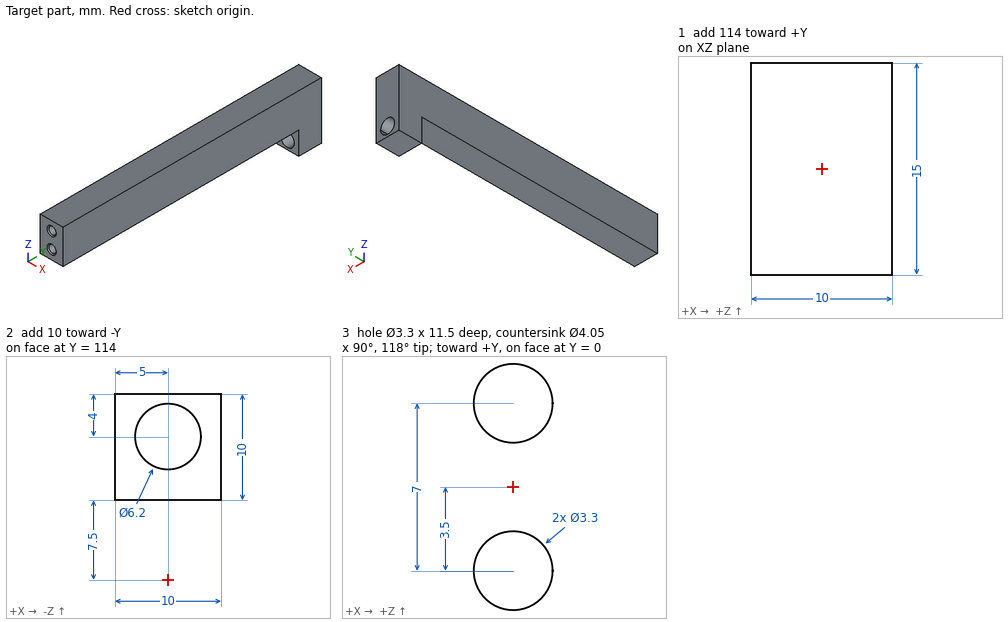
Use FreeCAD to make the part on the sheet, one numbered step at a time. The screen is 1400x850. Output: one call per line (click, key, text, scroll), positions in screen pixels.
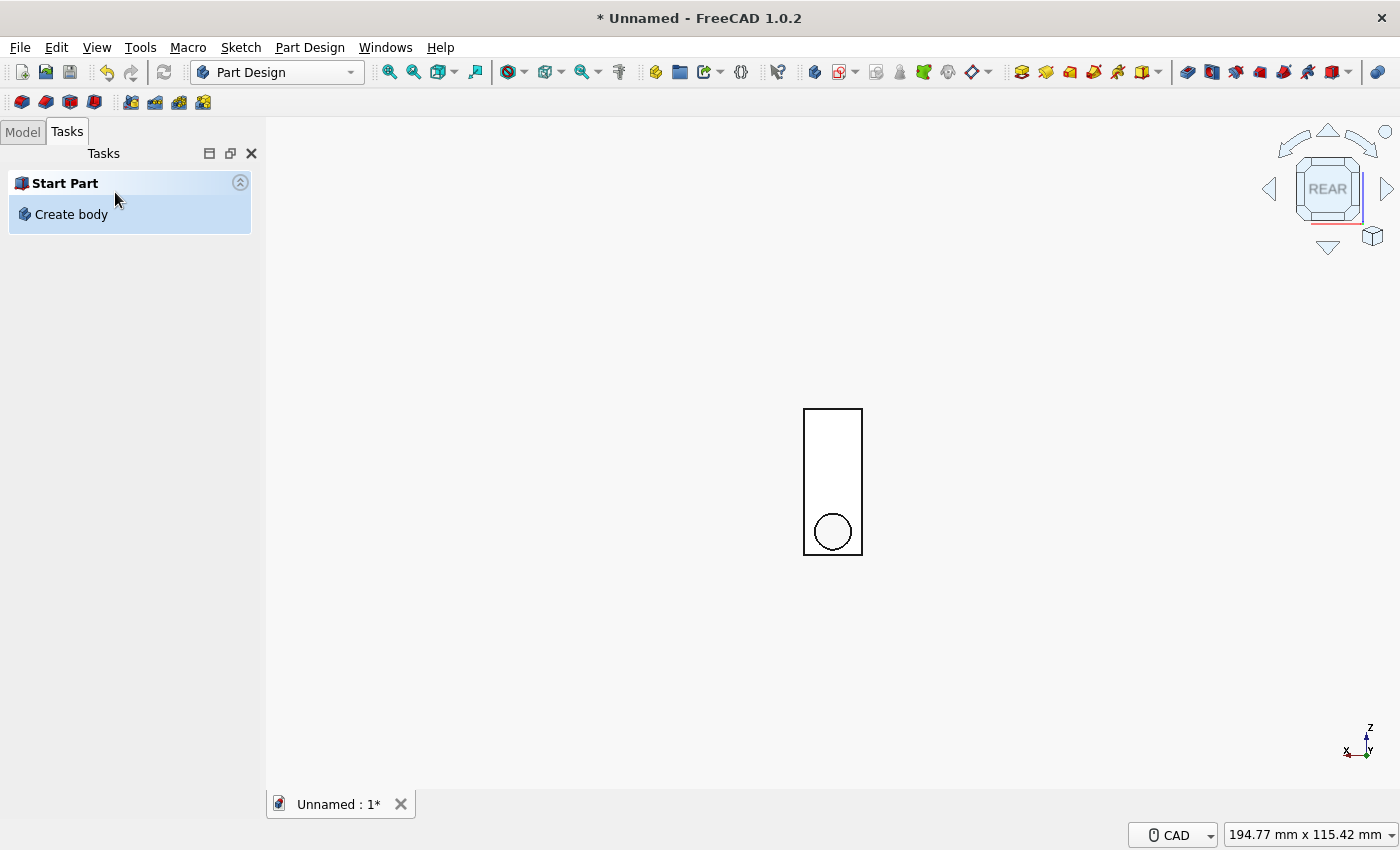
click(390, 72)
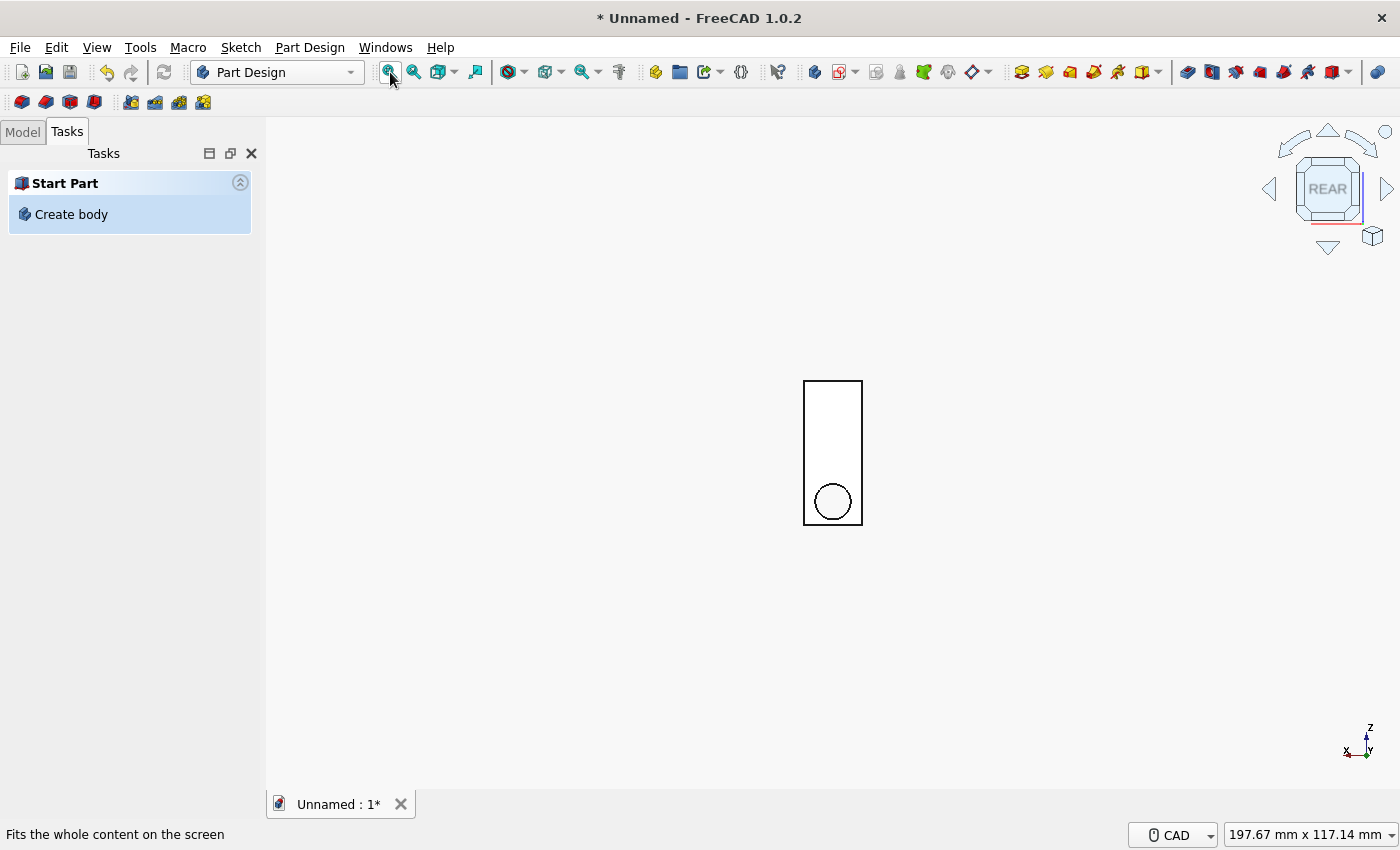
key(0)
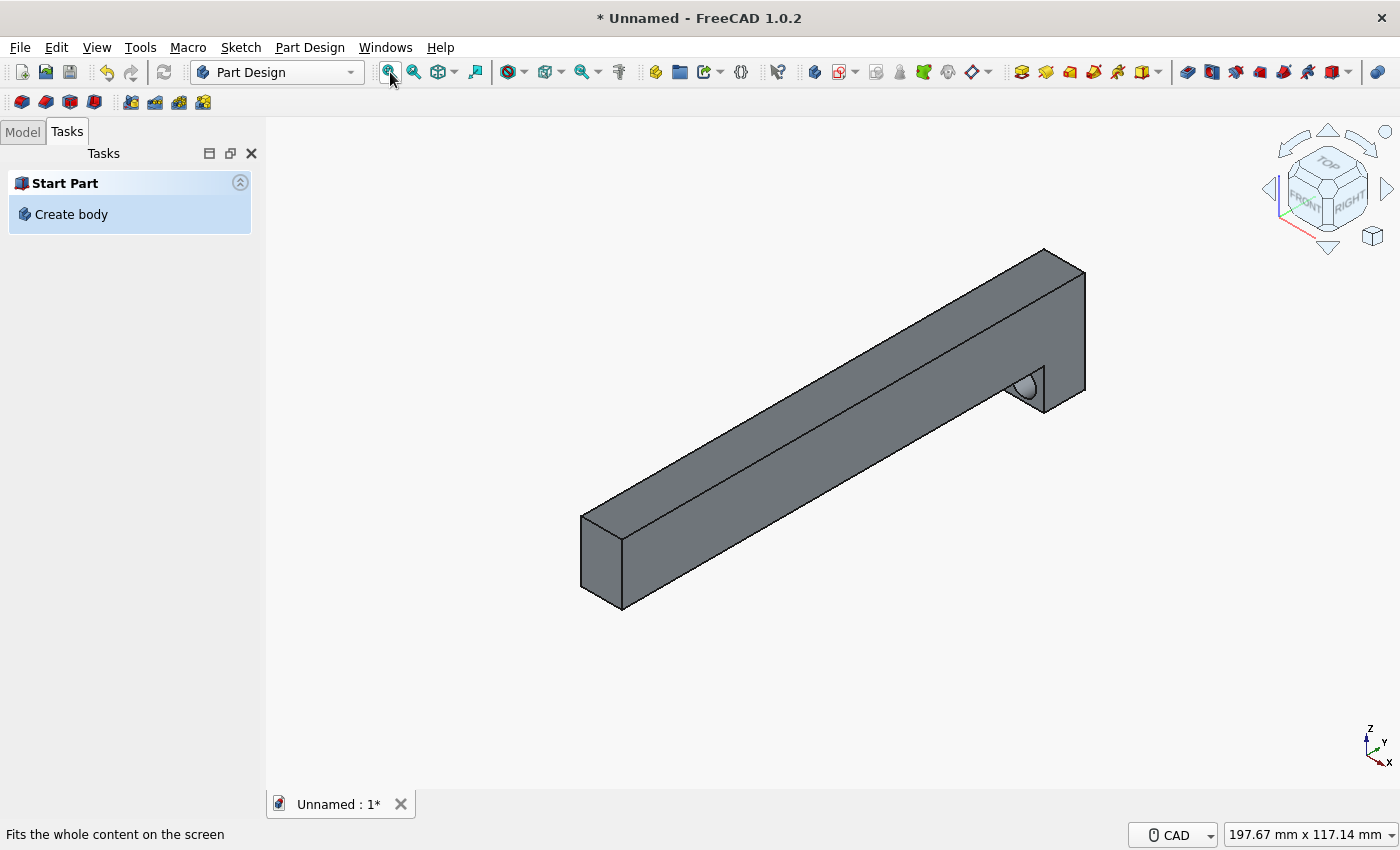
click(602, 552)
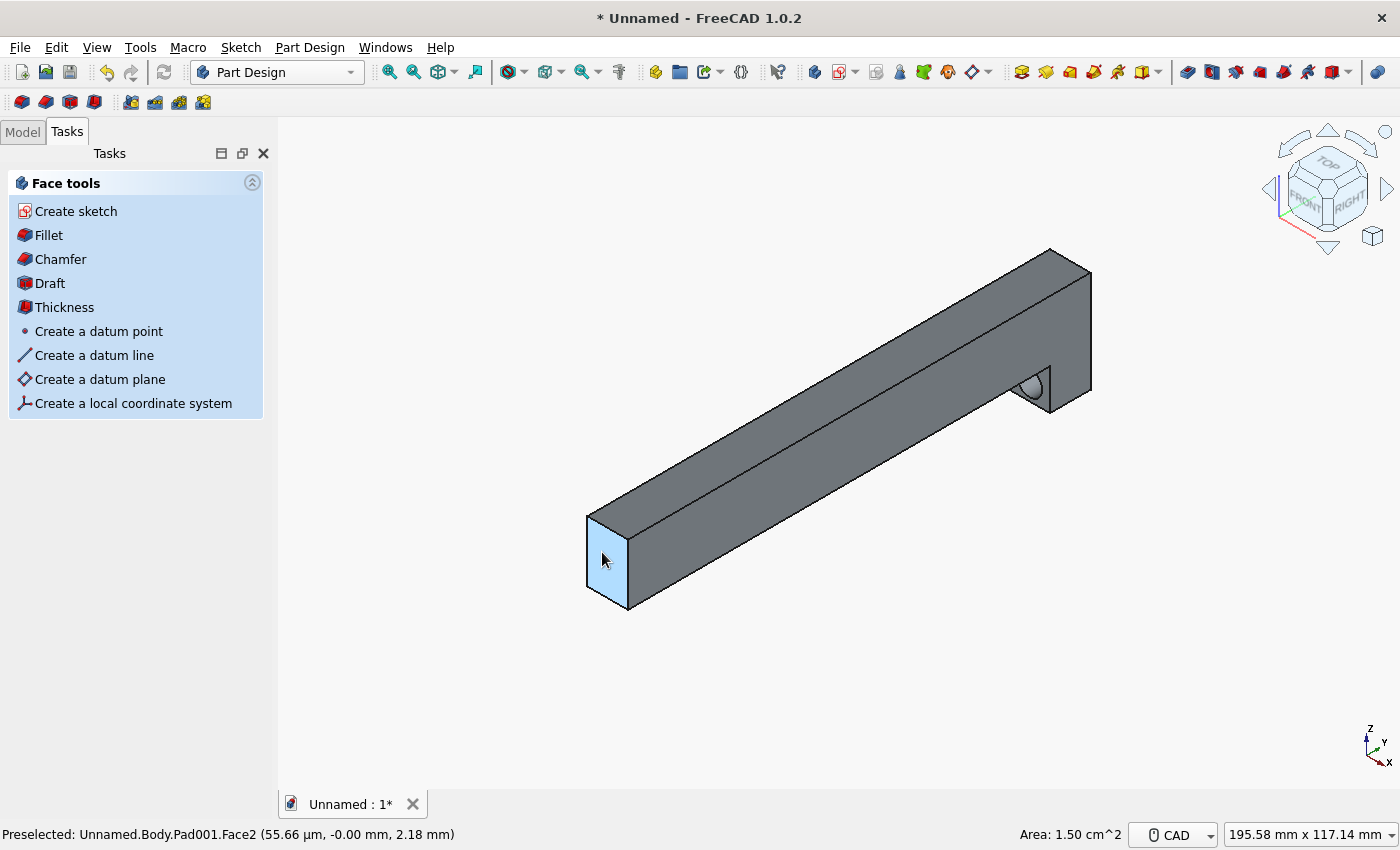
click(840, 72)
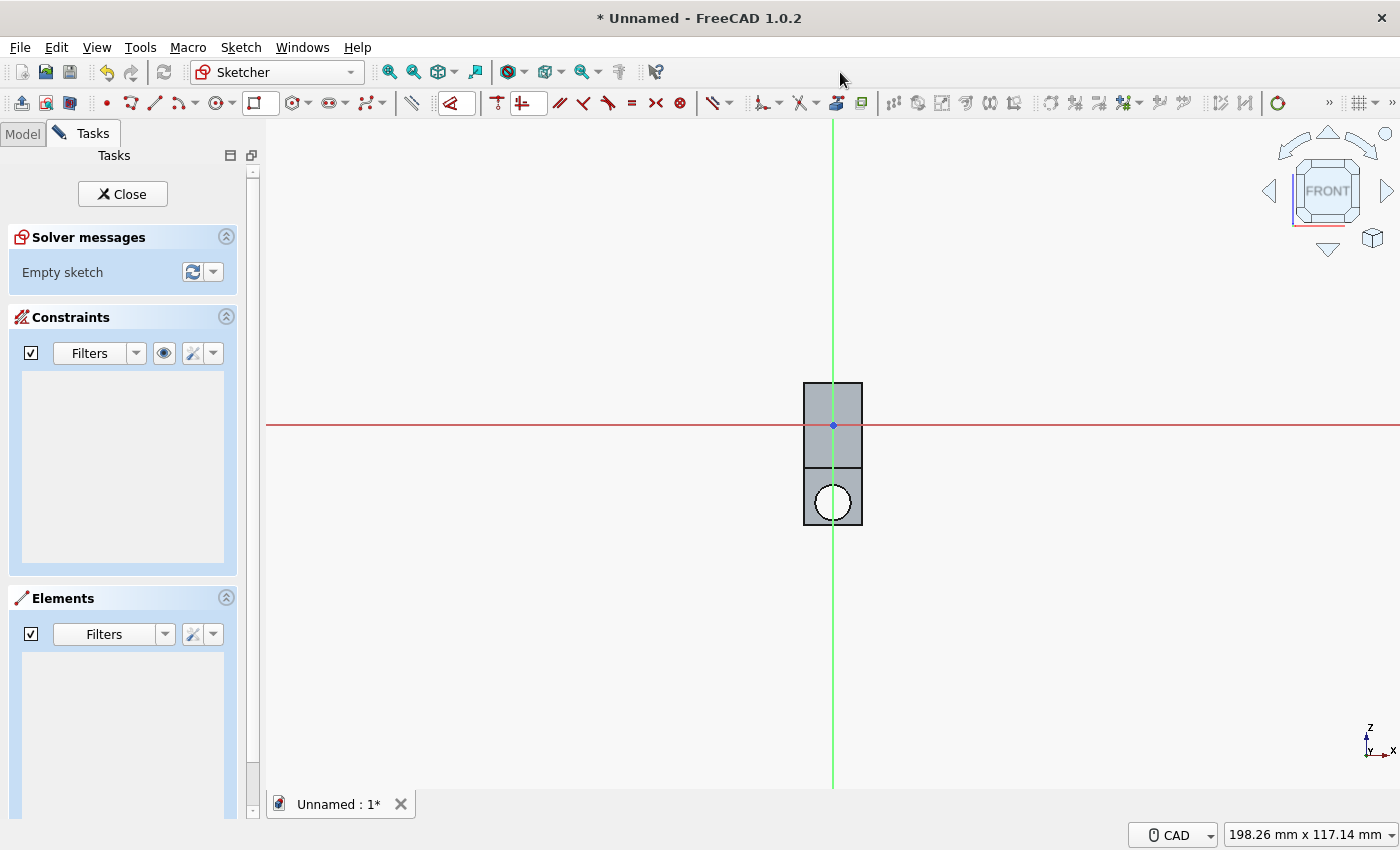
scroll(844, 421, up, 10)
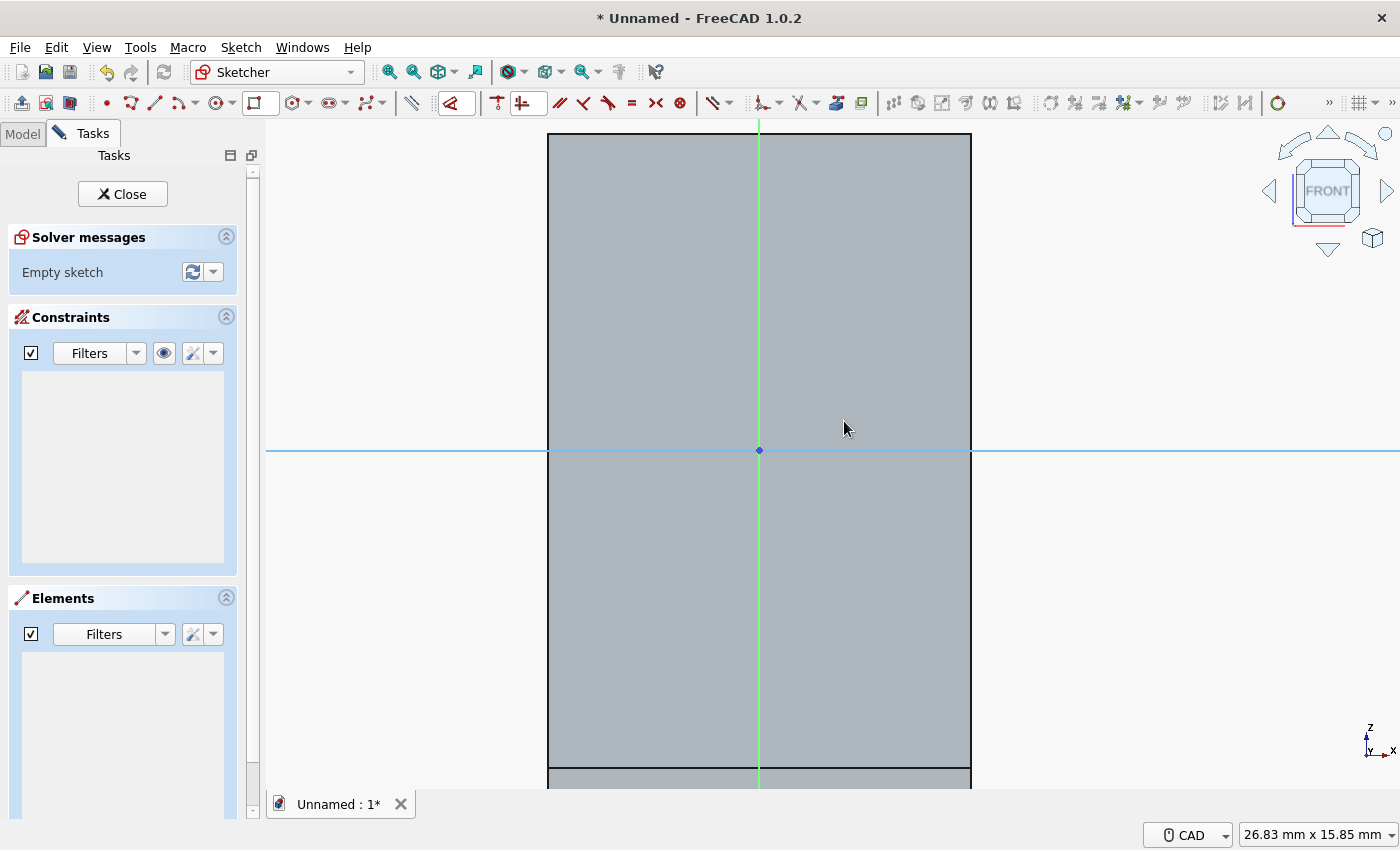
click(216, 104)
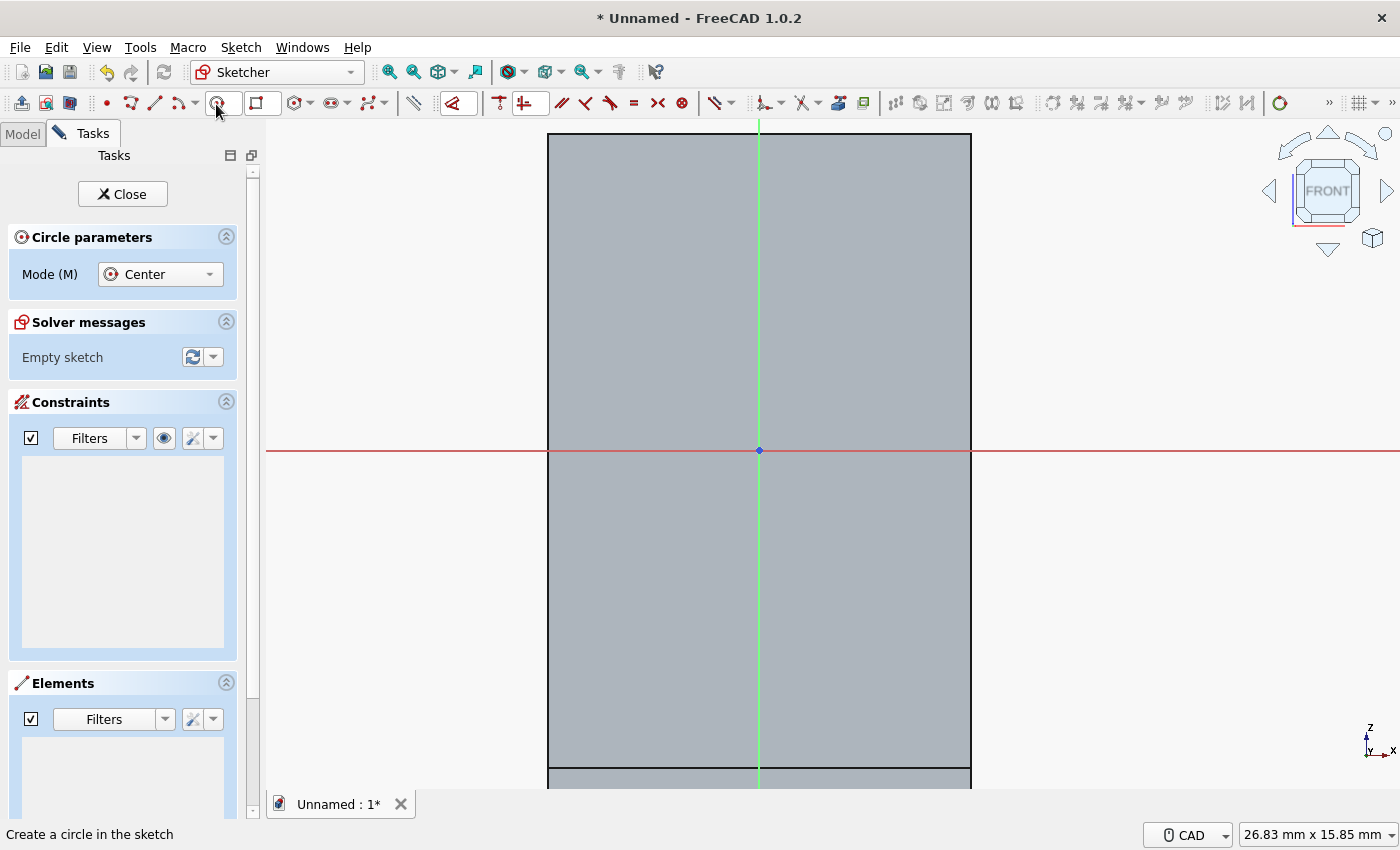
click(759, 599)
move(809, 549)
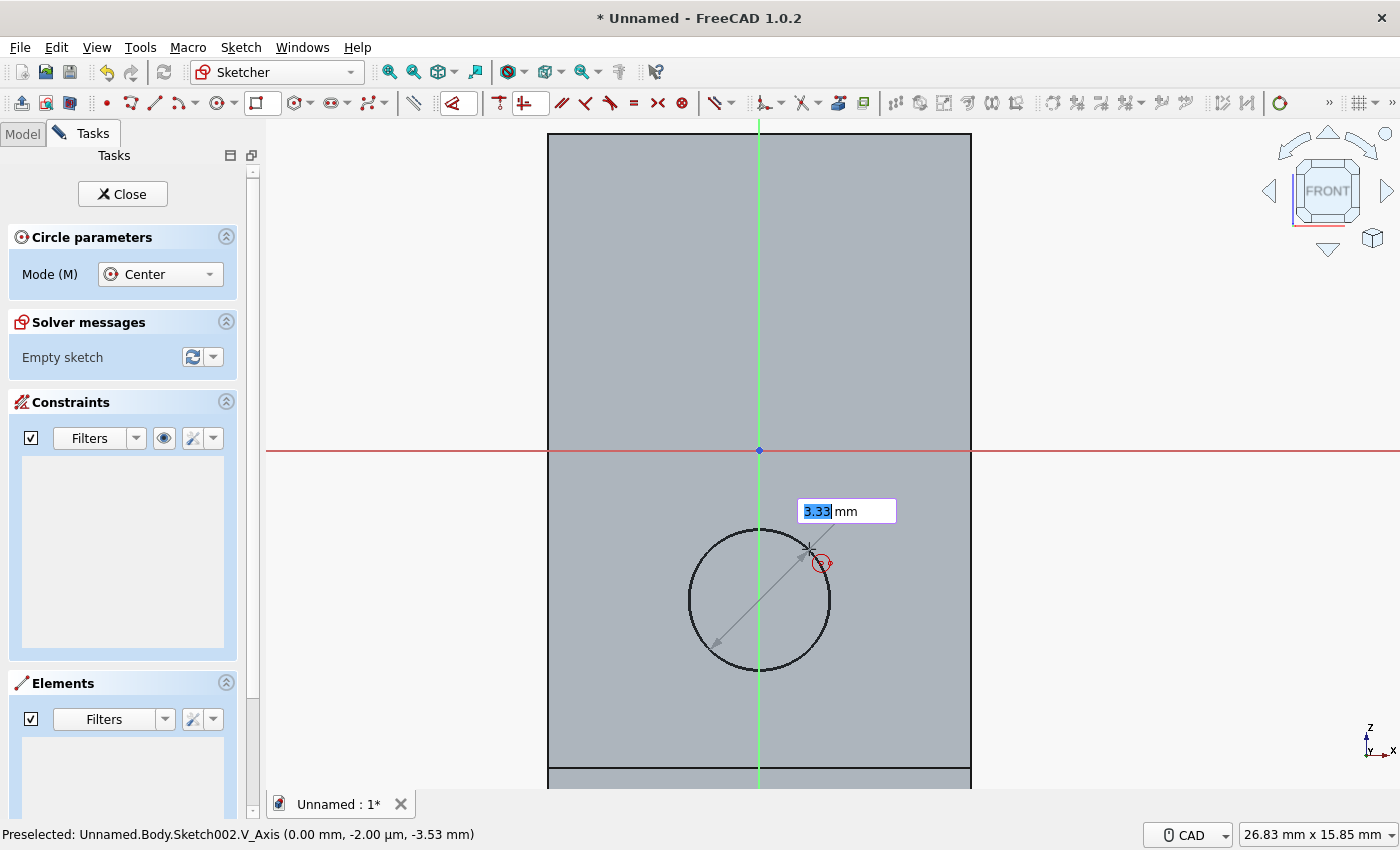
text(3.3)
key(Return)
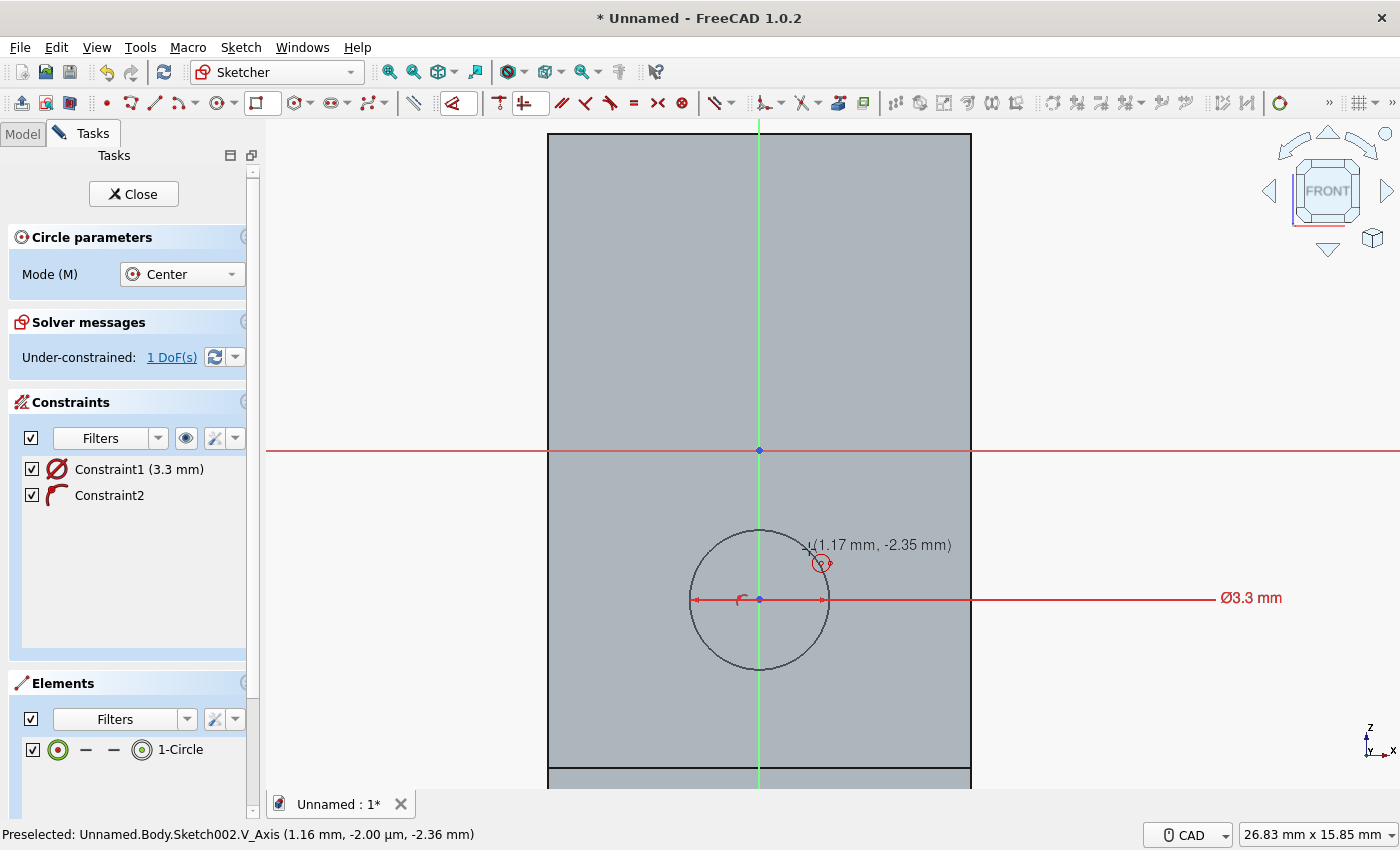
click(759, 303)
move(809, 253)